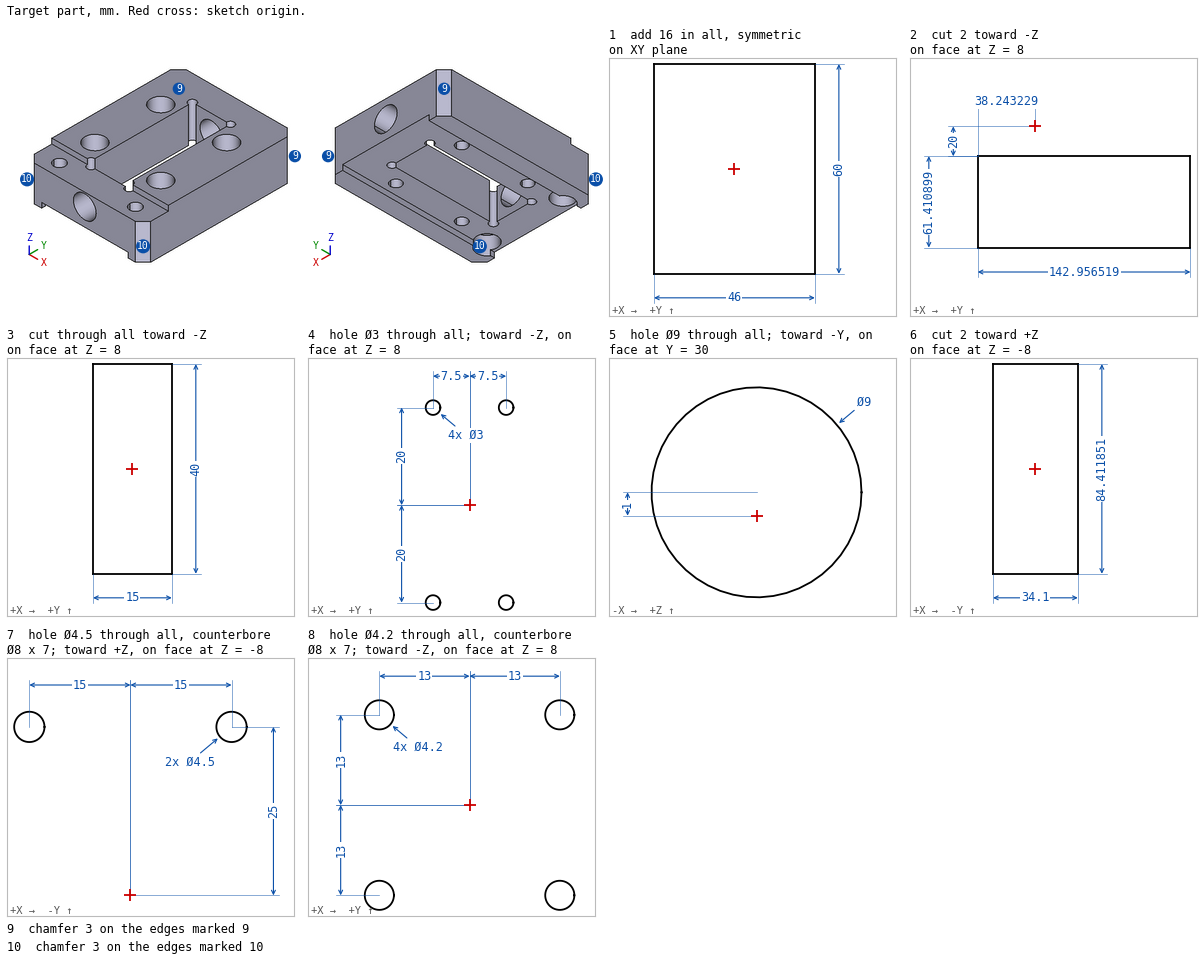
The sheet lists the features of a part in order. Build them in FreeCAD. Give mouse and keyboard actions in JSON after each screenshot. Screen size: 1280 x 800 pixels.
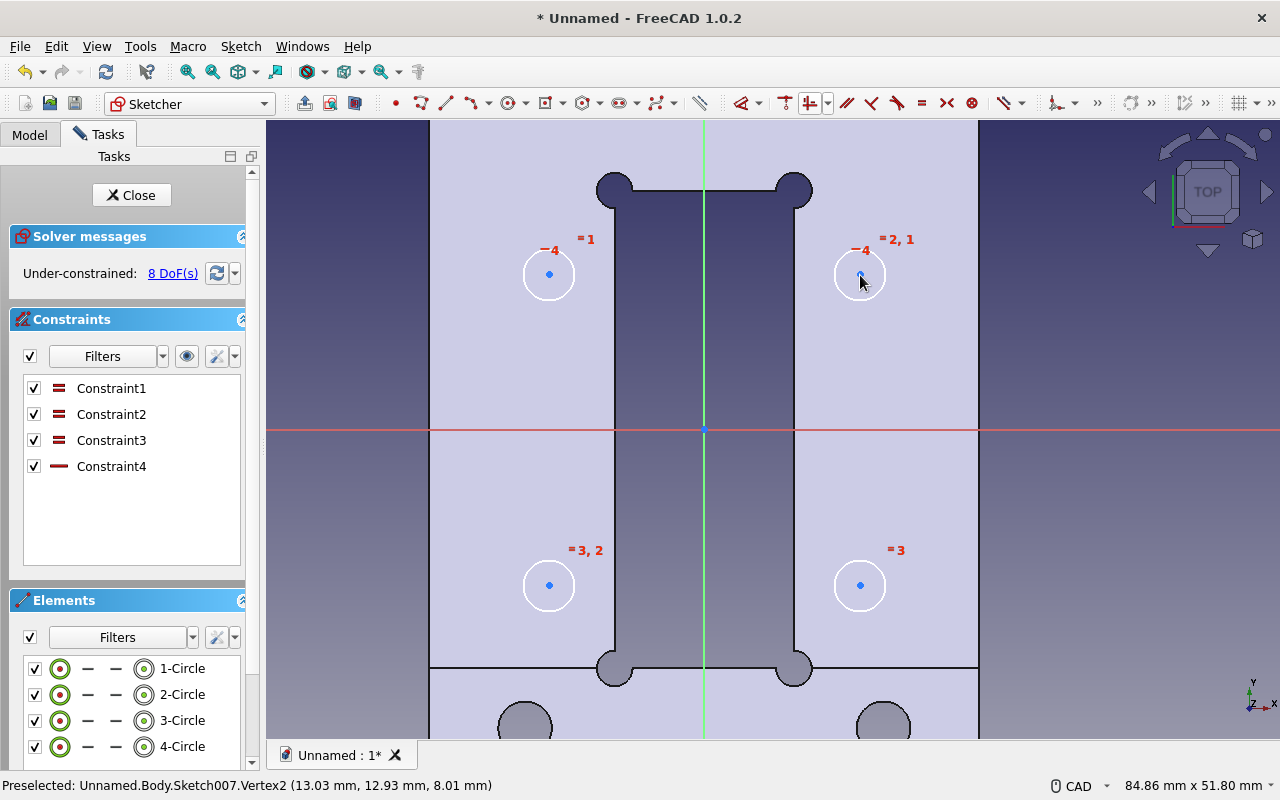
{"action": "left_click", "coordinate": [549, 275]}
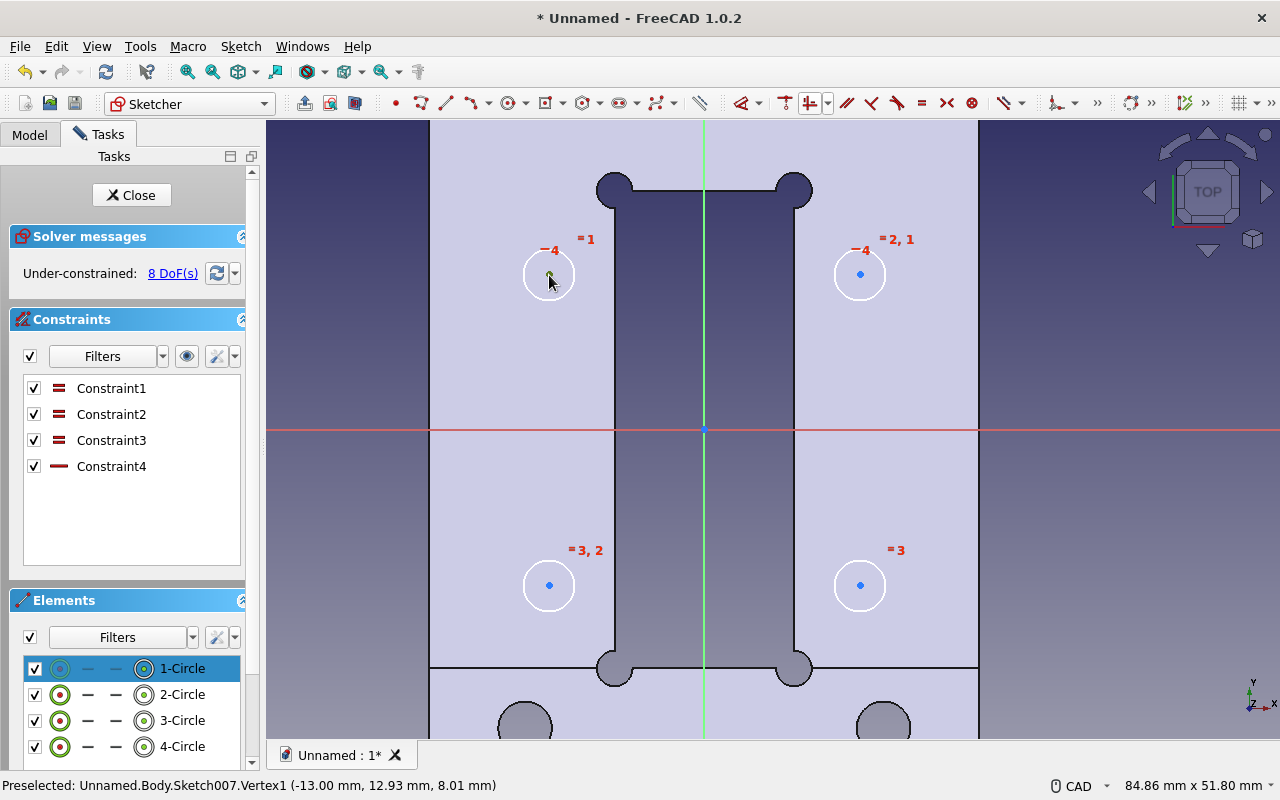
{"action": "left_click", "coordinate": [549, 586]}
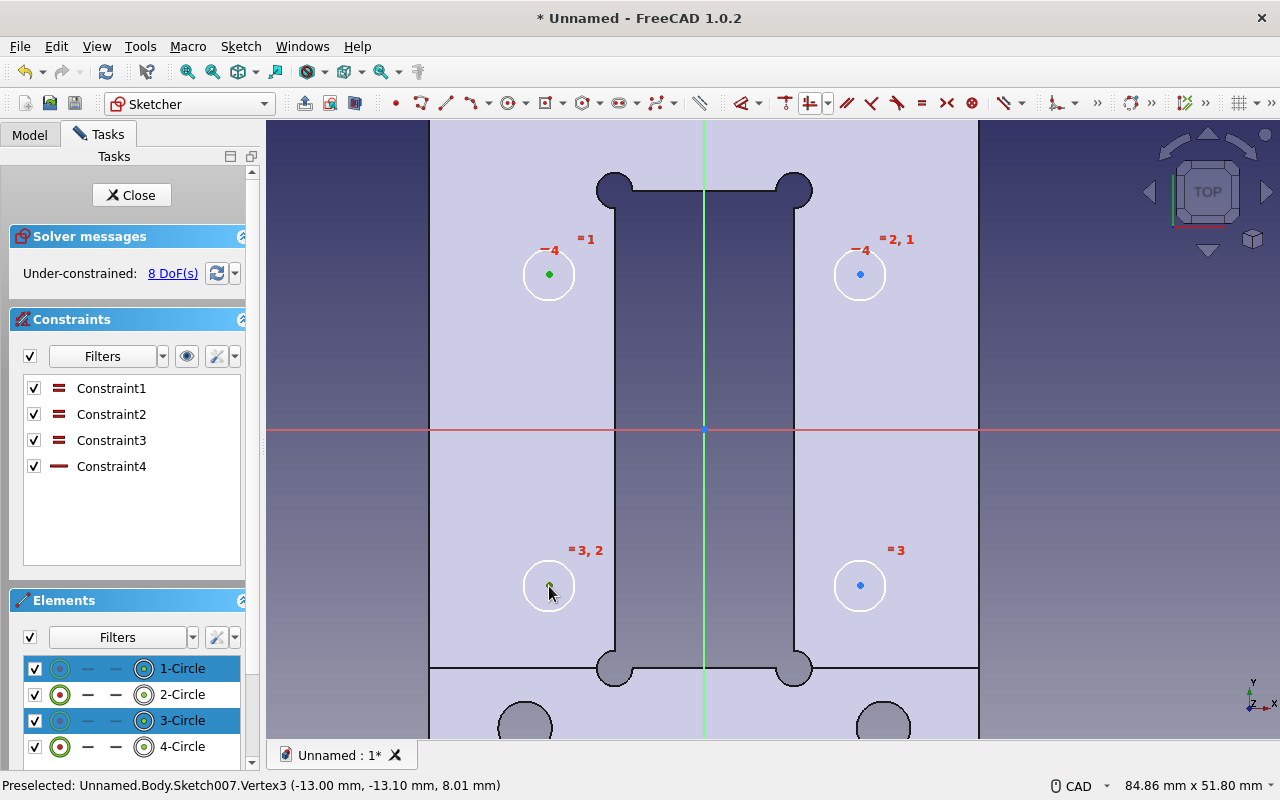
{"action": "key", "text": "v"}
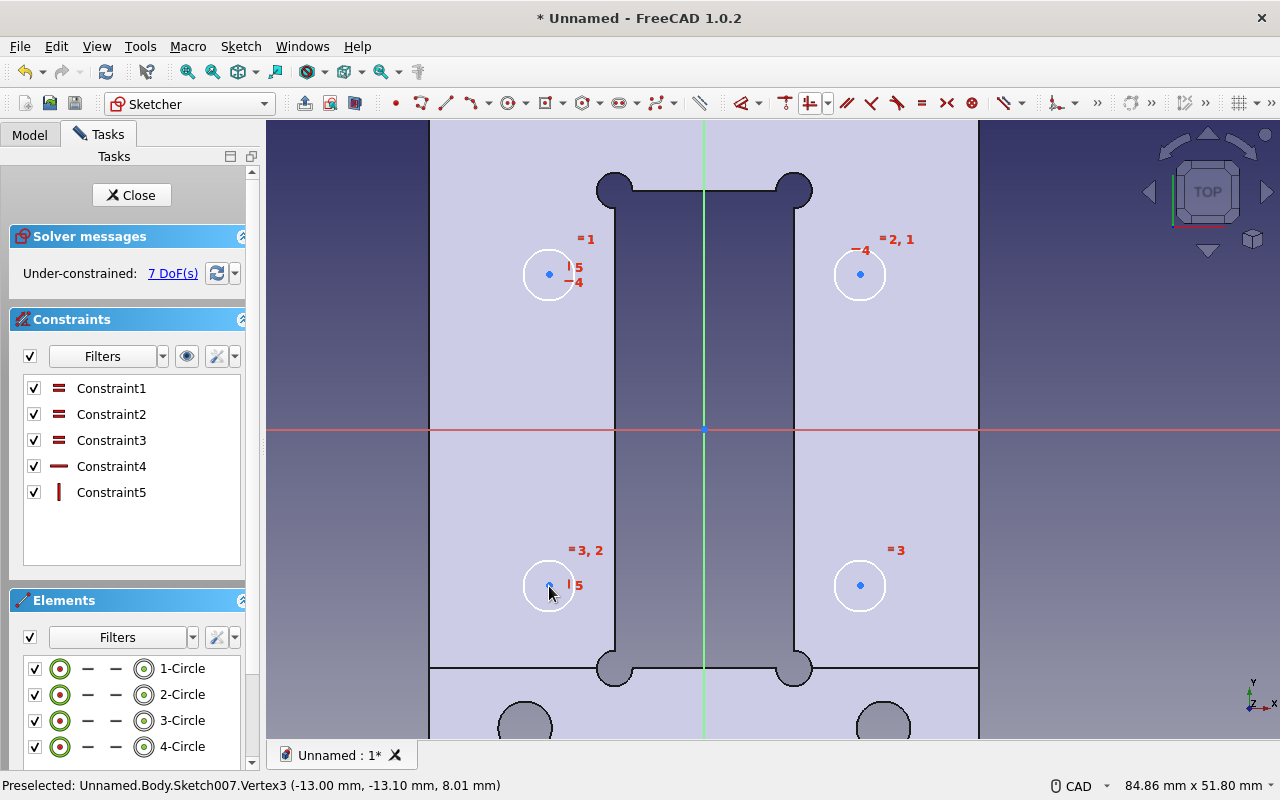
{"action": "left_click", "coordinate": [860, 275]}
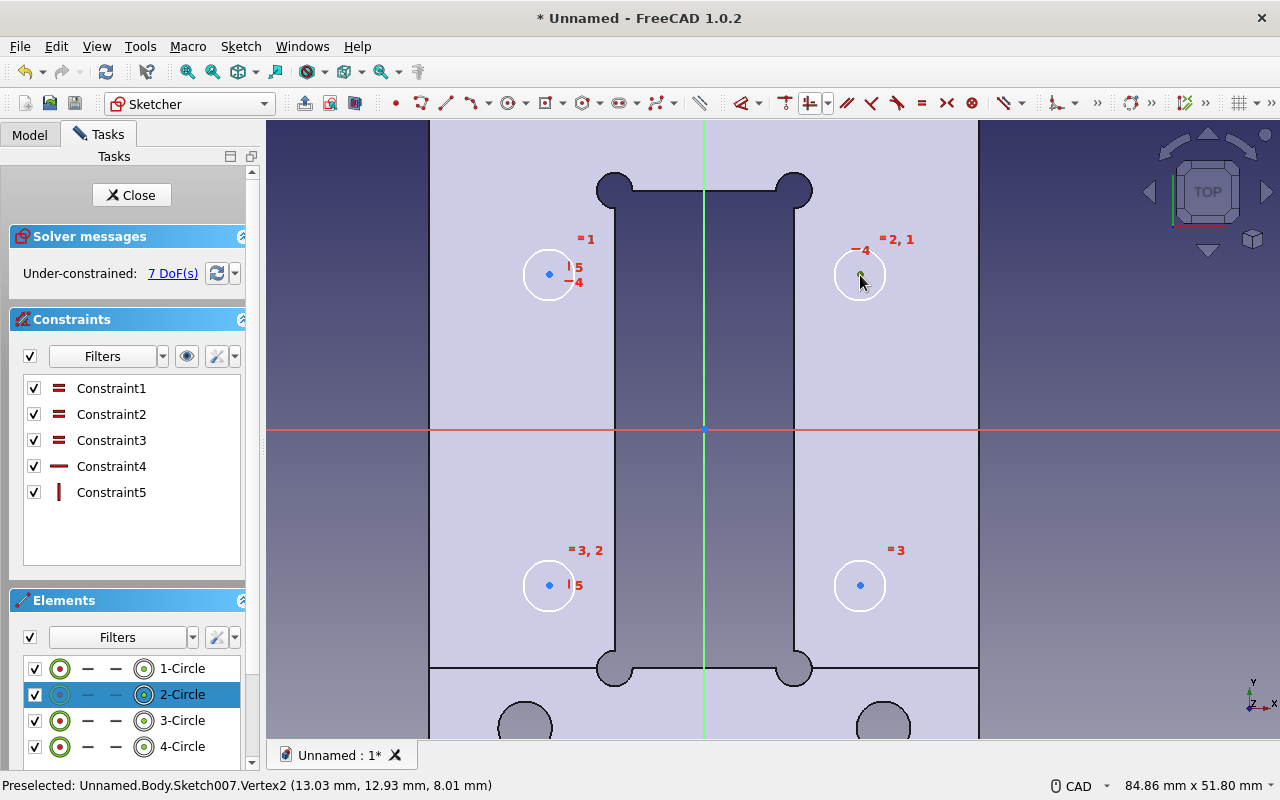
{"action": "left_click", "coordinate": [860, 586]}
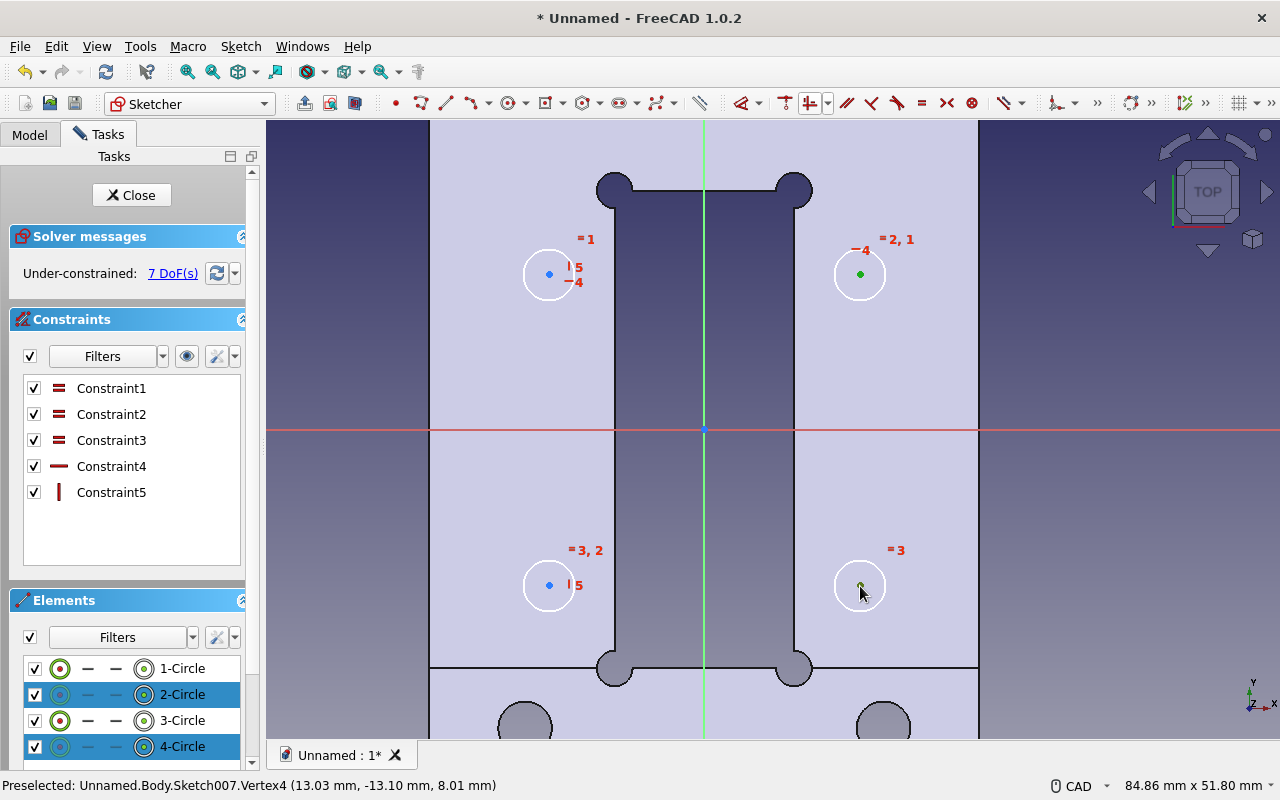
{"action": "left_click", "coordinate": [828, 104]}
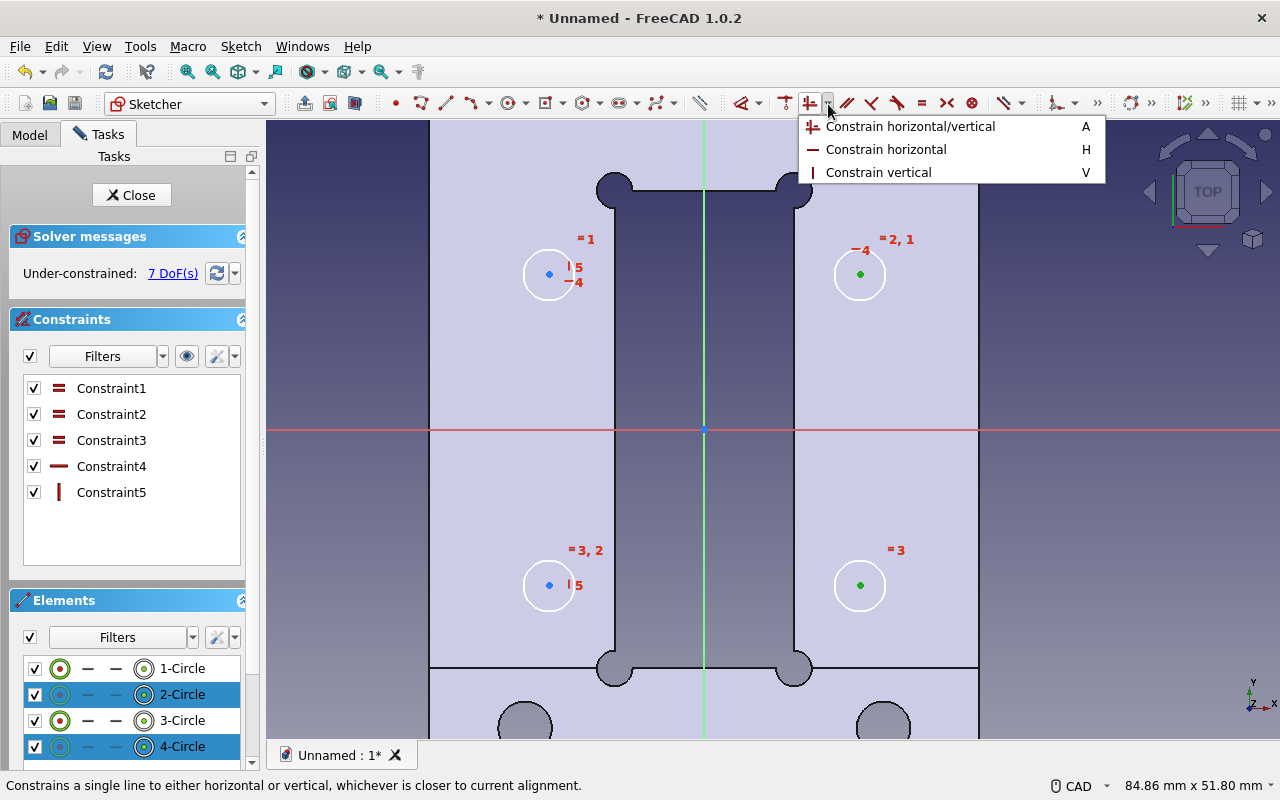
{"action": "left_click", "coordinate": [952, 172]}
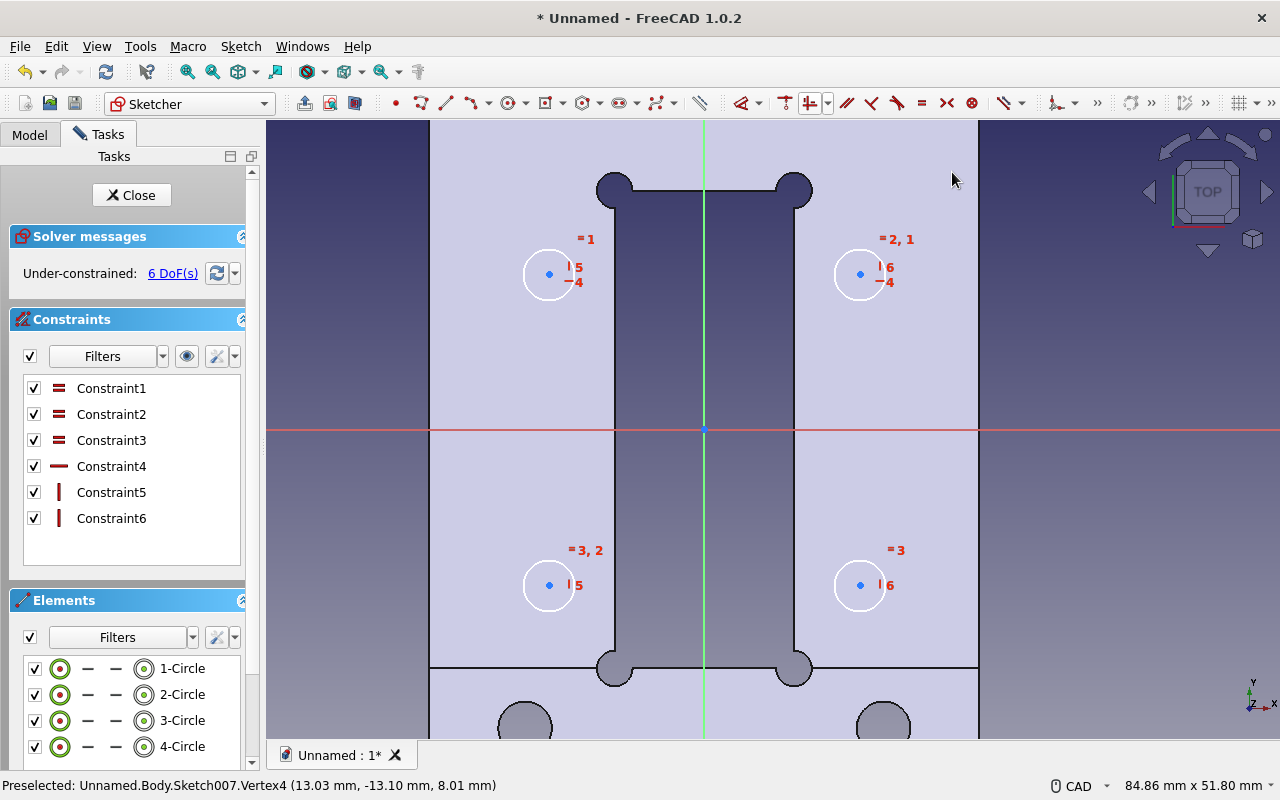
{"action": "left_click", "coordinate": [549, 586]}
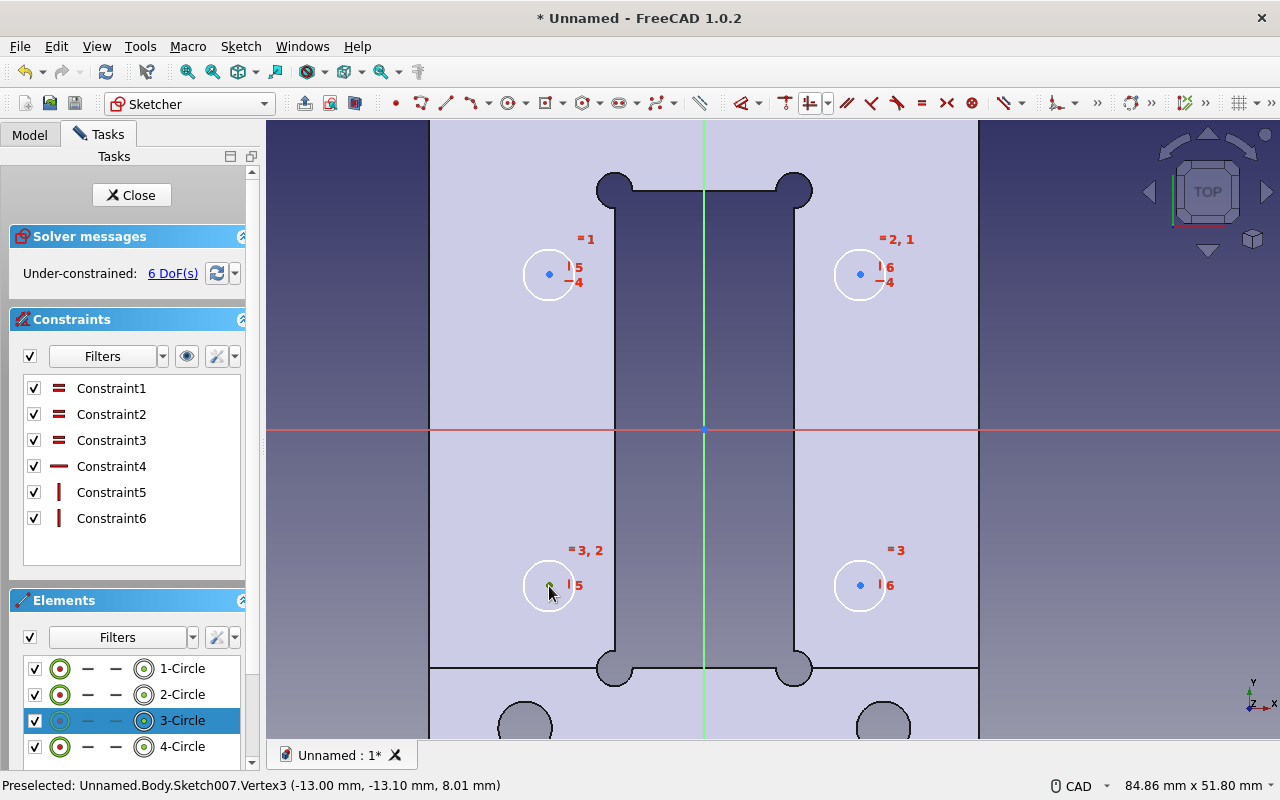
{"action": "left_click", "coordinate": [860, 586]}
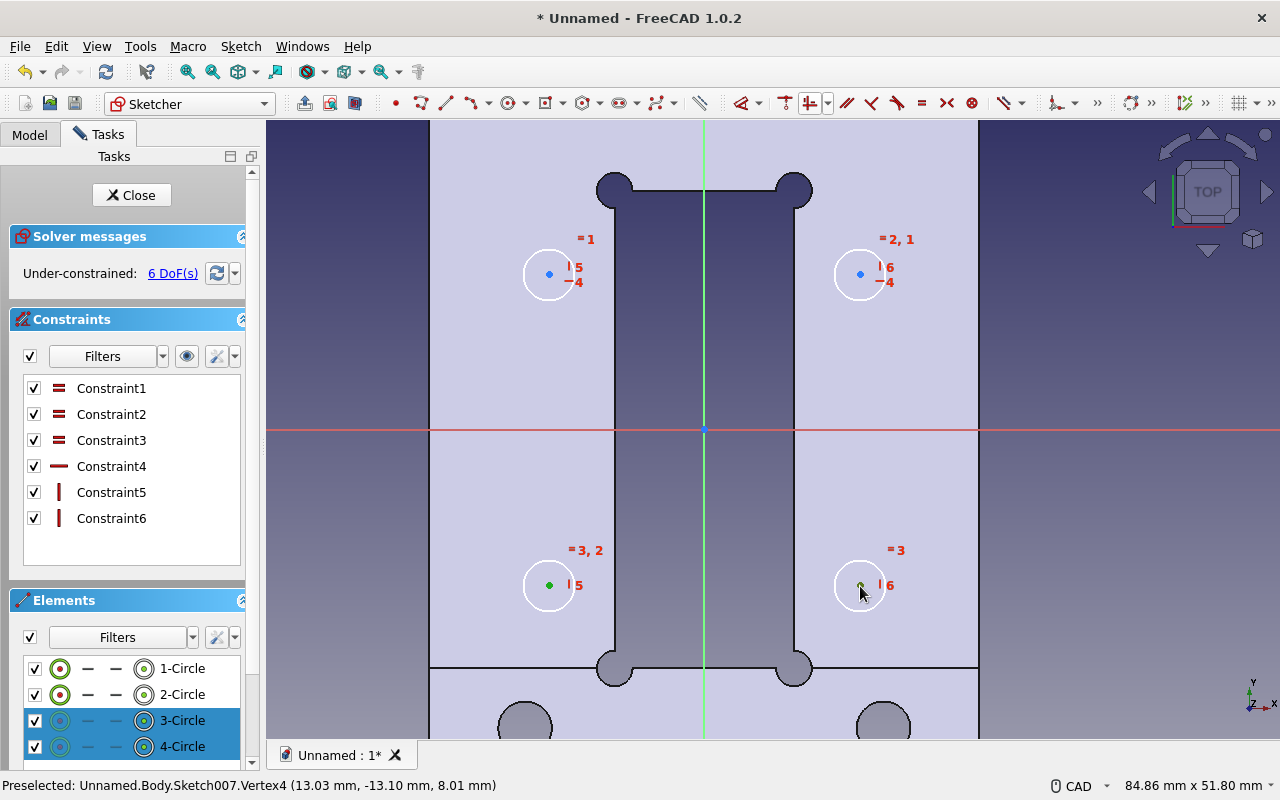
{"action": "key", "text": "h"}